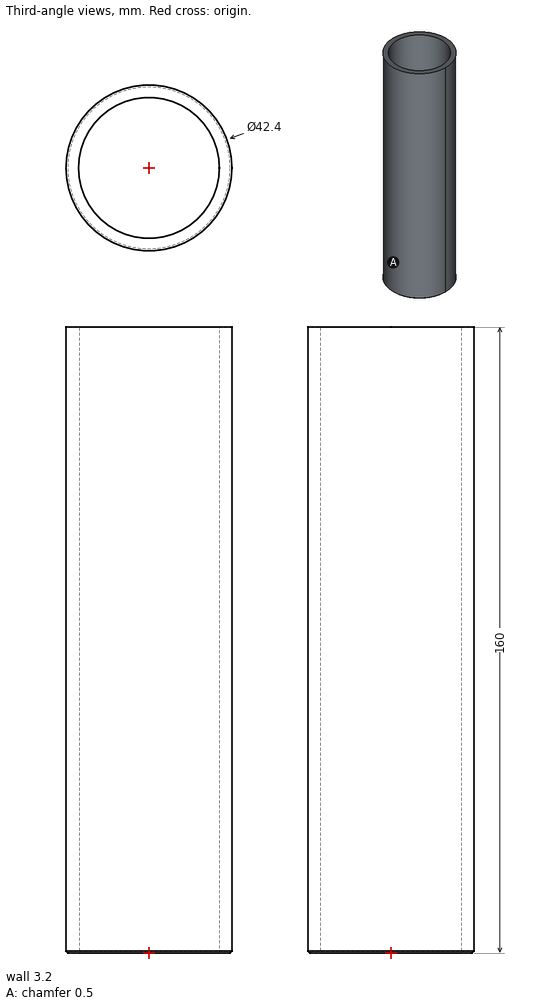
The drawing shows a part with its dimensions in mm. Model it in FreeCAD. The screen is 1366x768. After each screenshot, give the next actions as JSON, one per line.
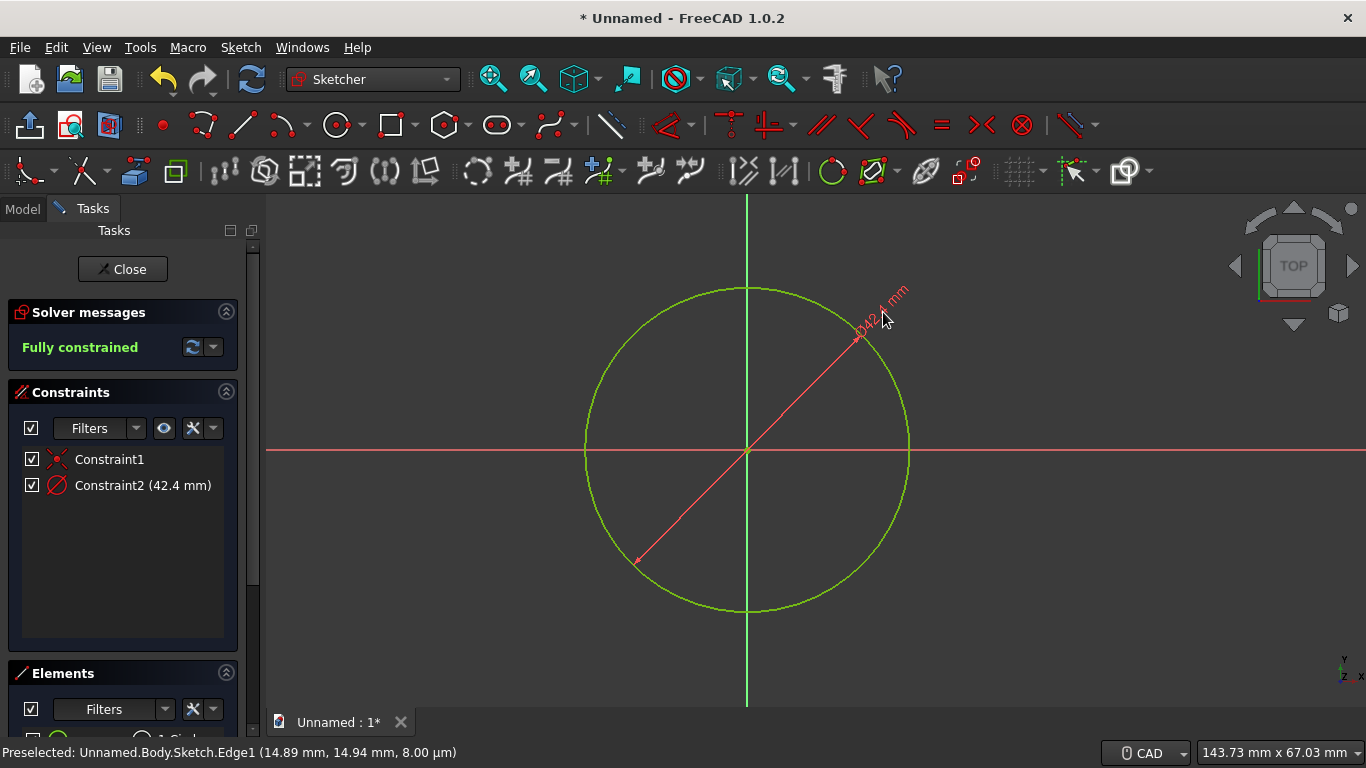
{"action": "left_click", "coordinate": [123, 269]}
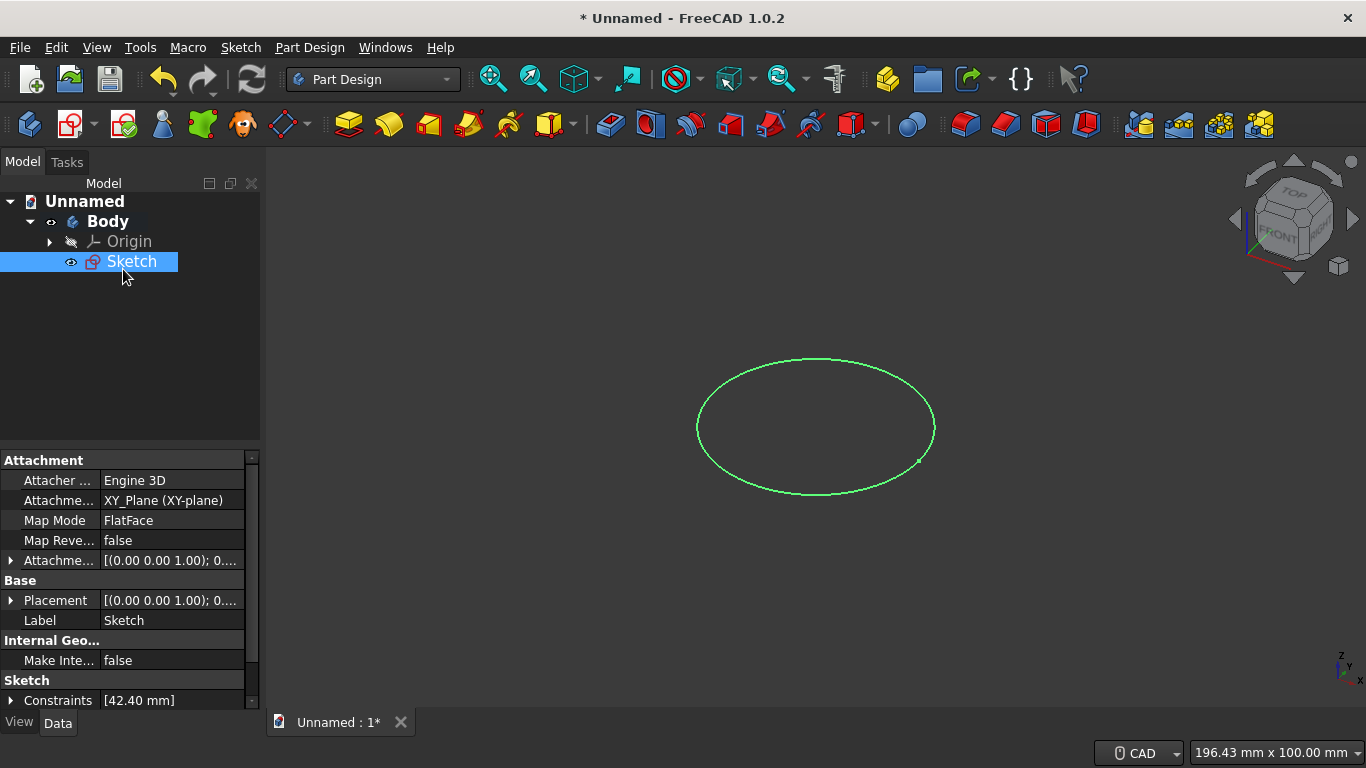
{"action": "left_click", "coordinate": [350, 124]}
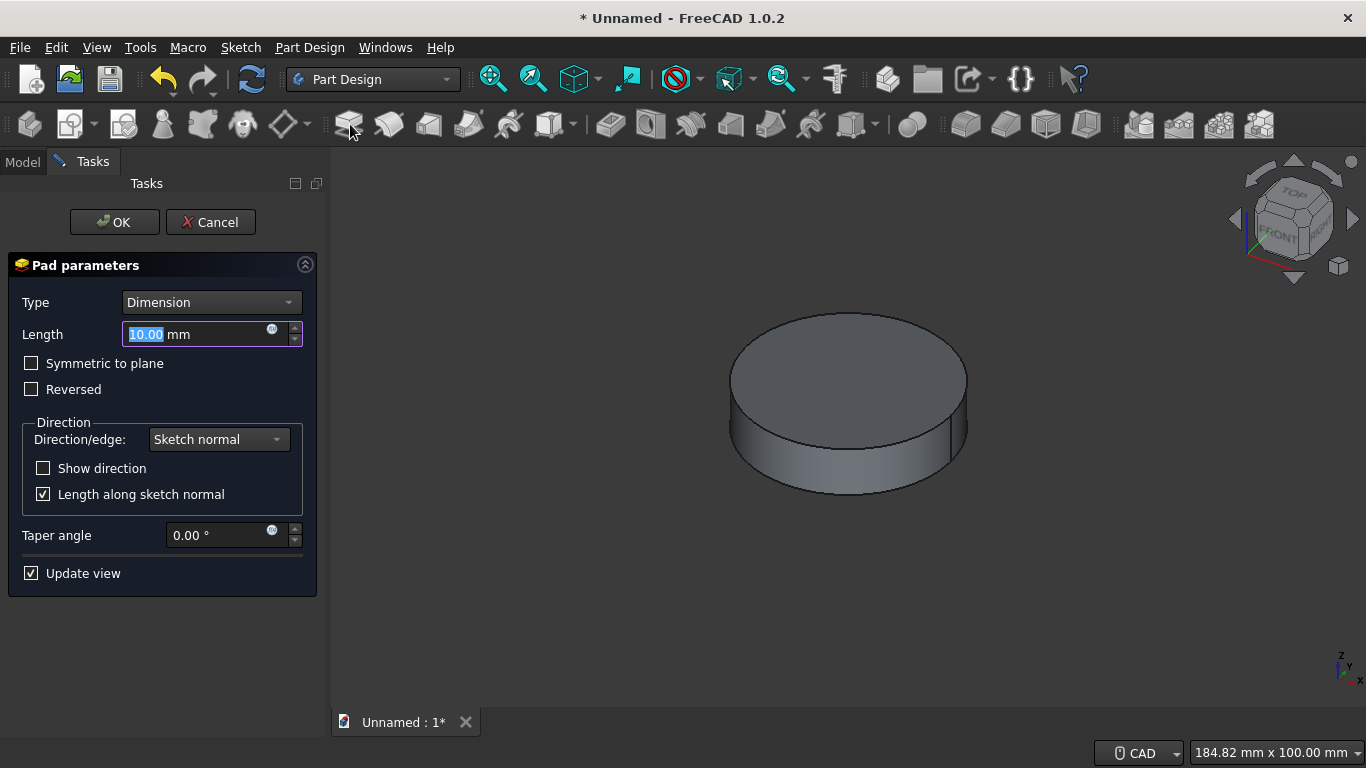
{"action": "type", "text": "160"}
{"action": "key", "text": "Tab"}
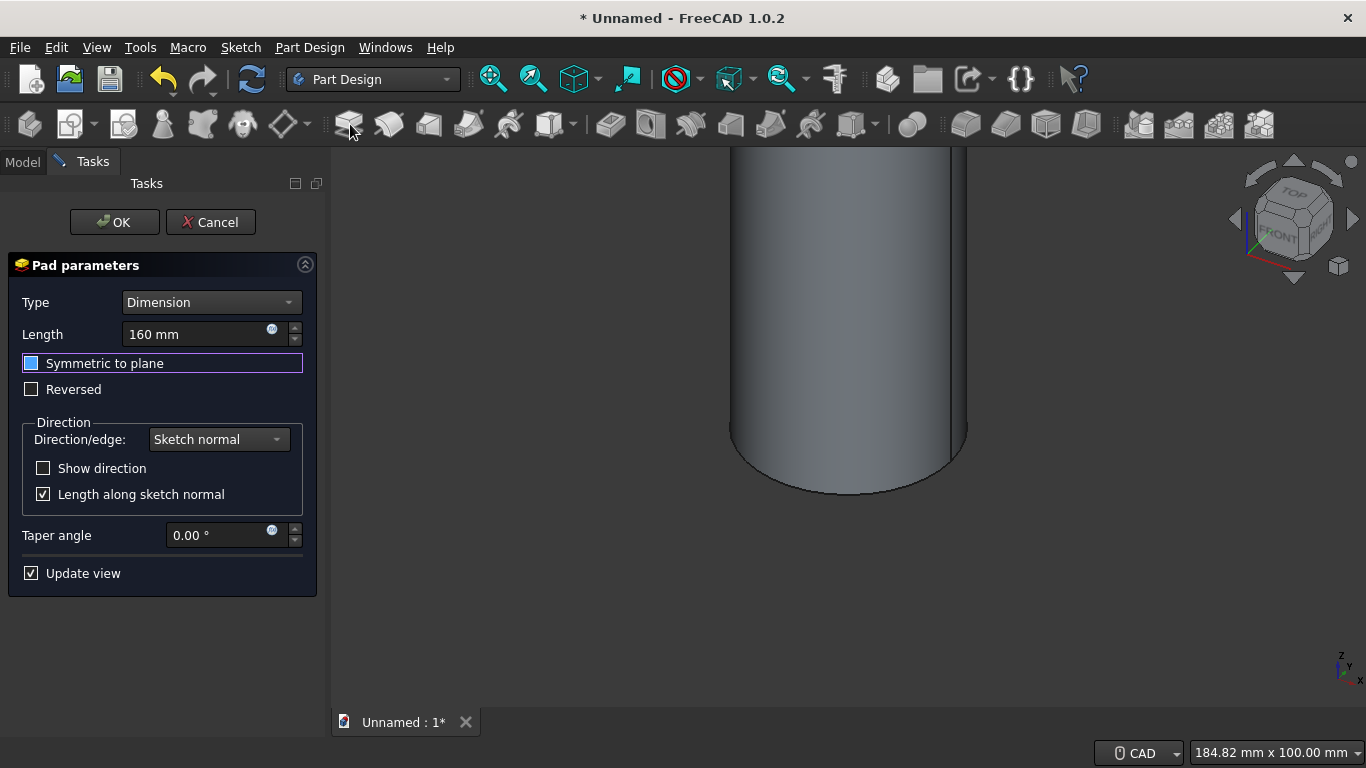
{"action": "left_click", "coordinate": [115, 222]}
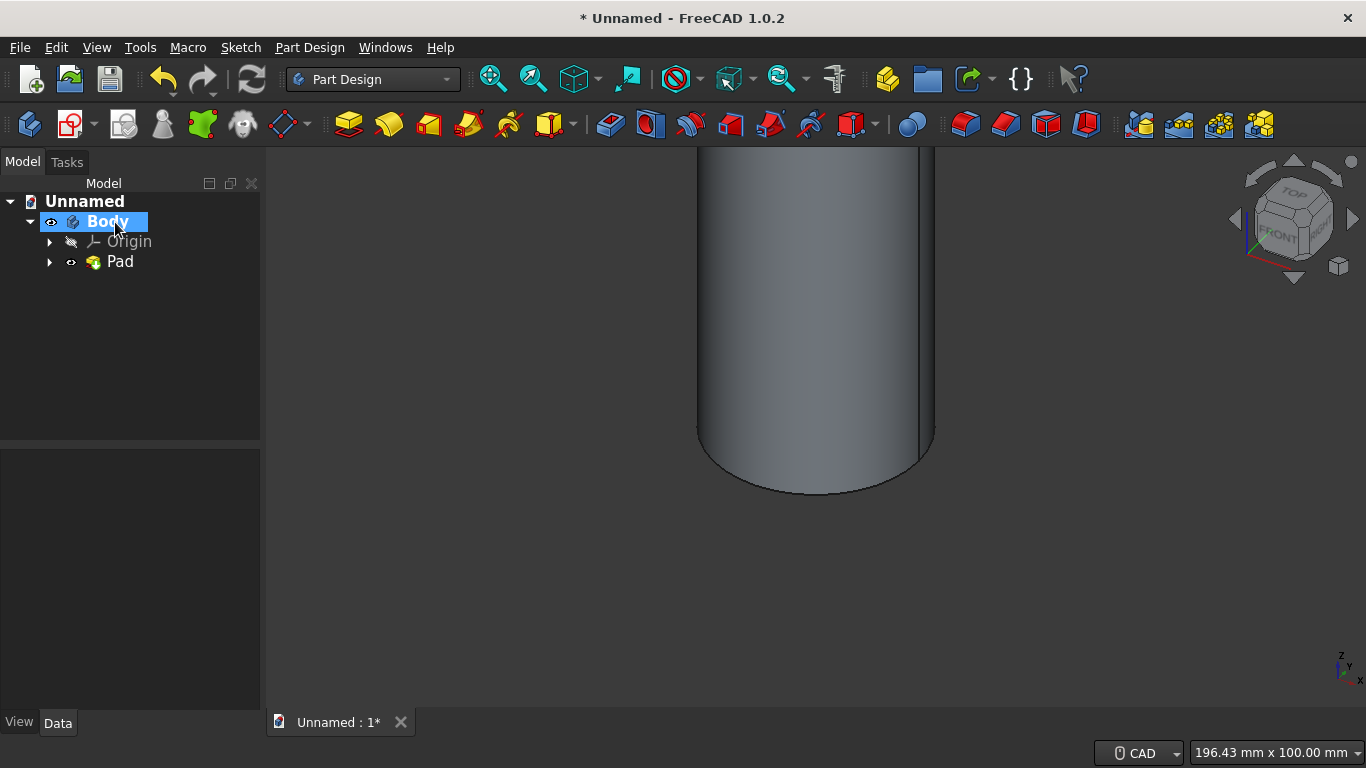
{"action": "left_click", "coordinate": [494, 80]}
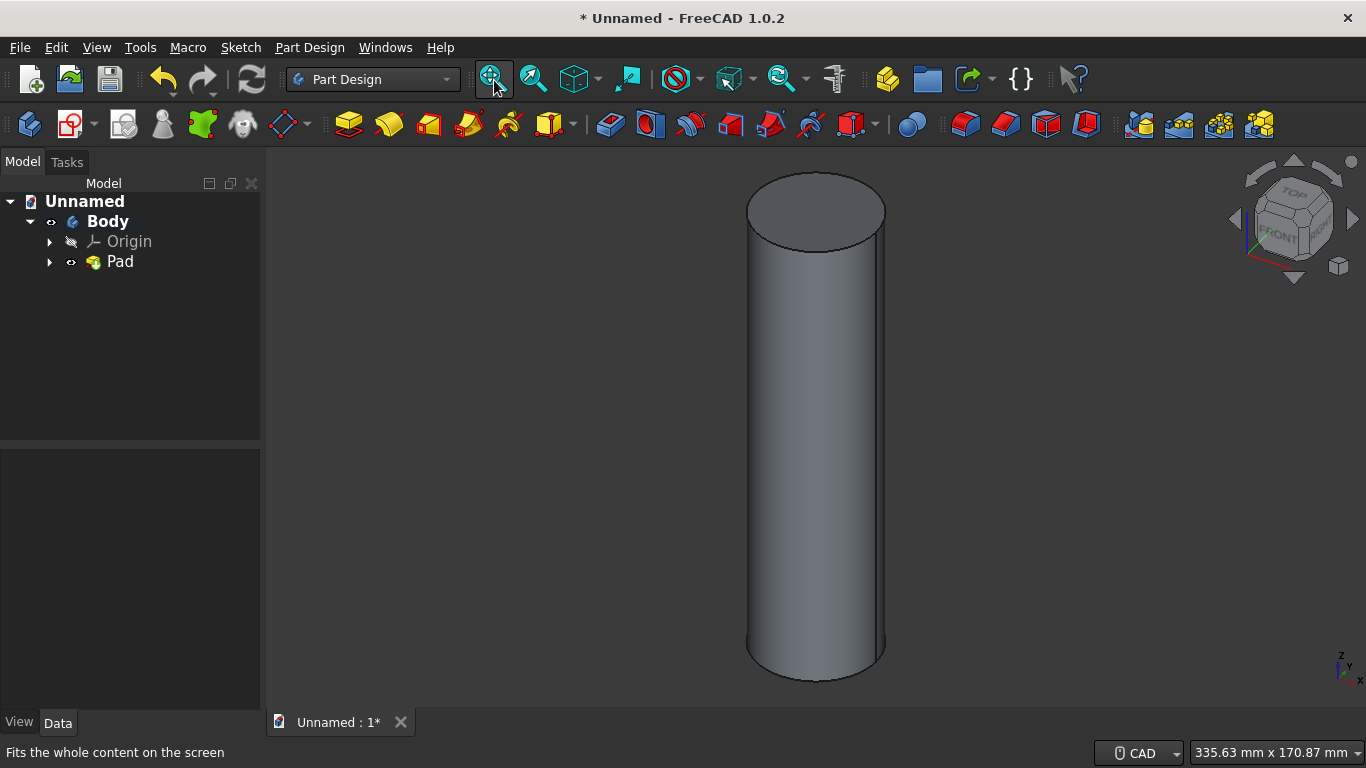
{"action": "left_click", "coordinate": [816, 211]}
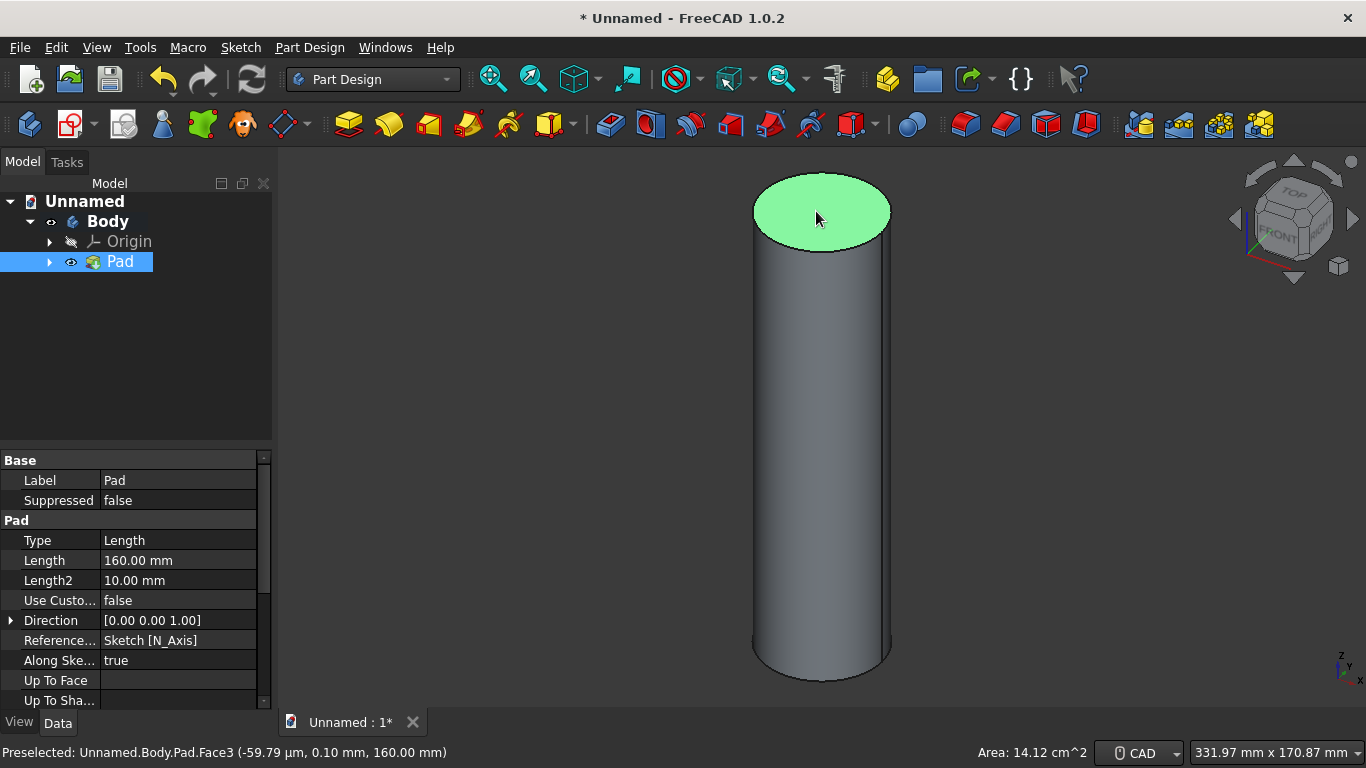
{"action": "key", "text": "0"}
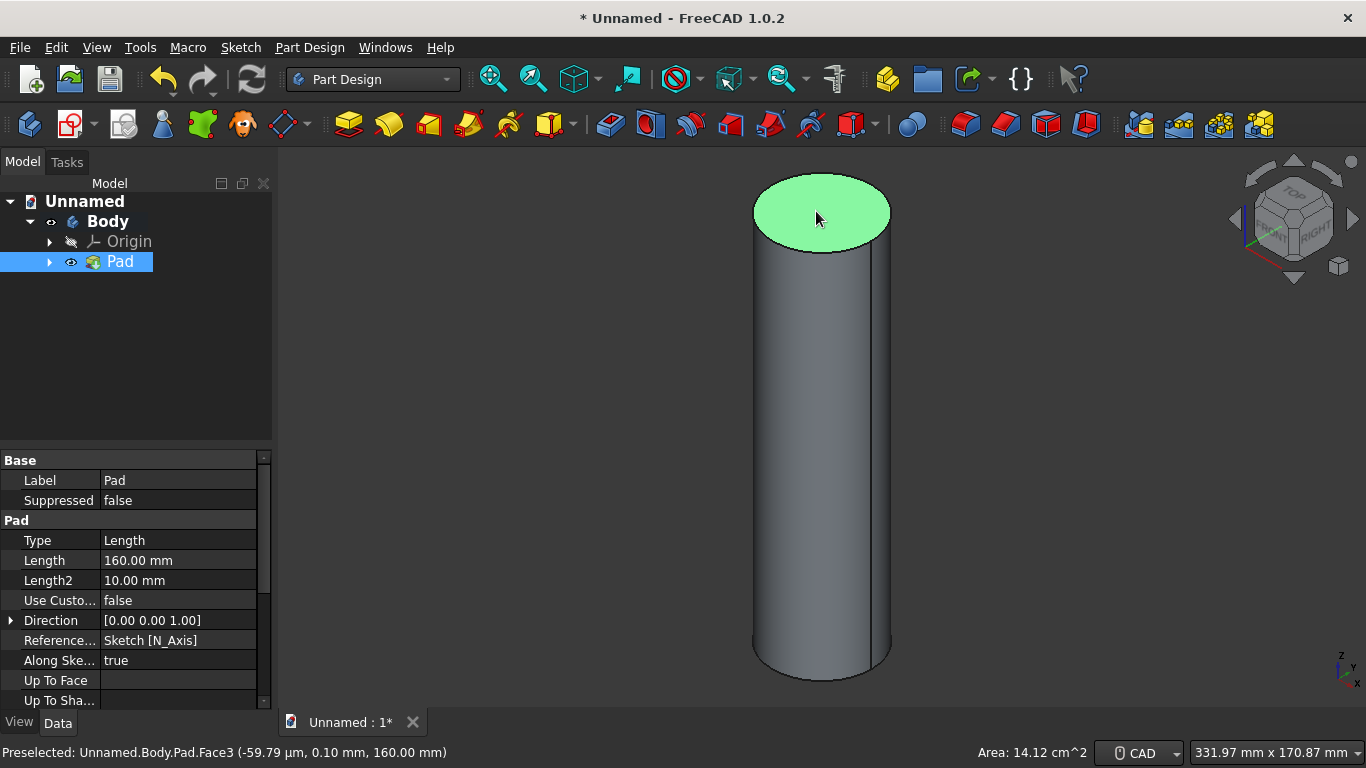
{"action": "key", "text": "2"}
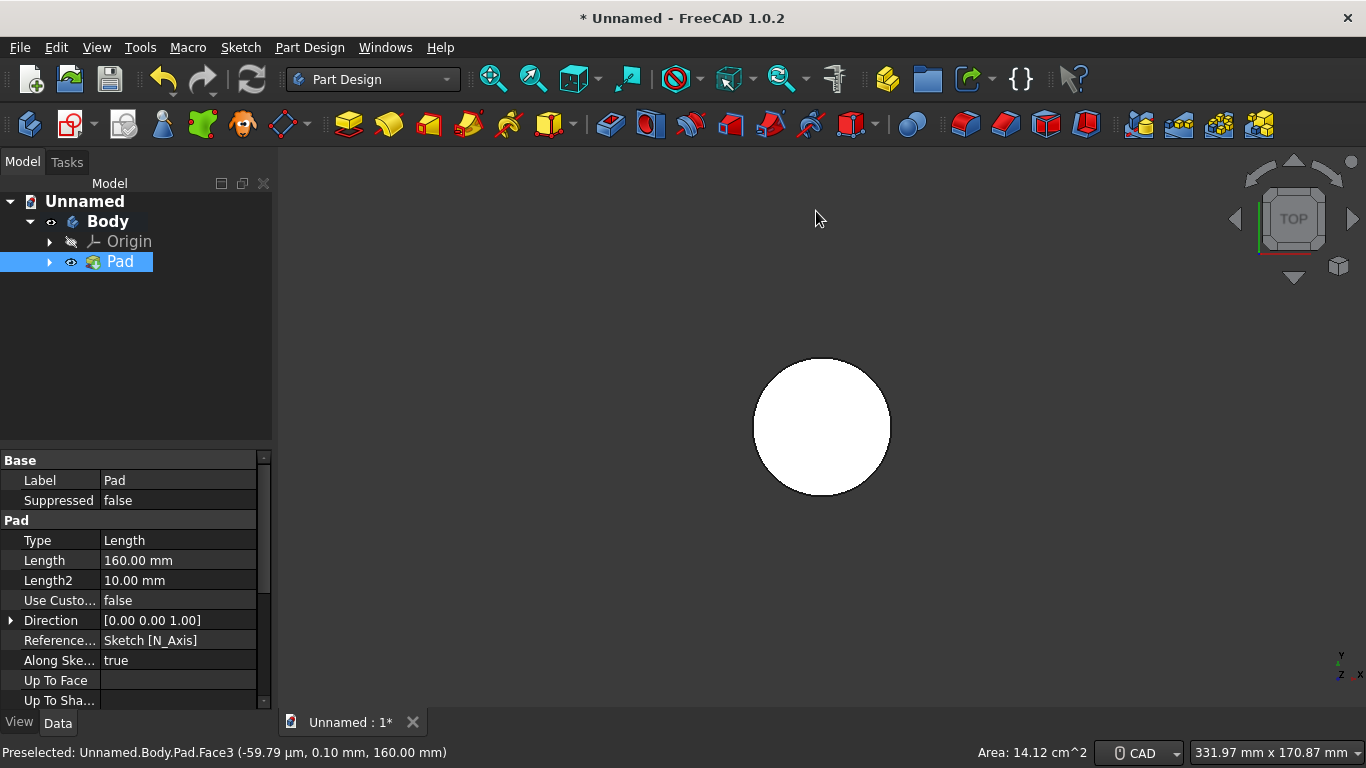
{"action": "left_click", "coordinate": [494, 80]}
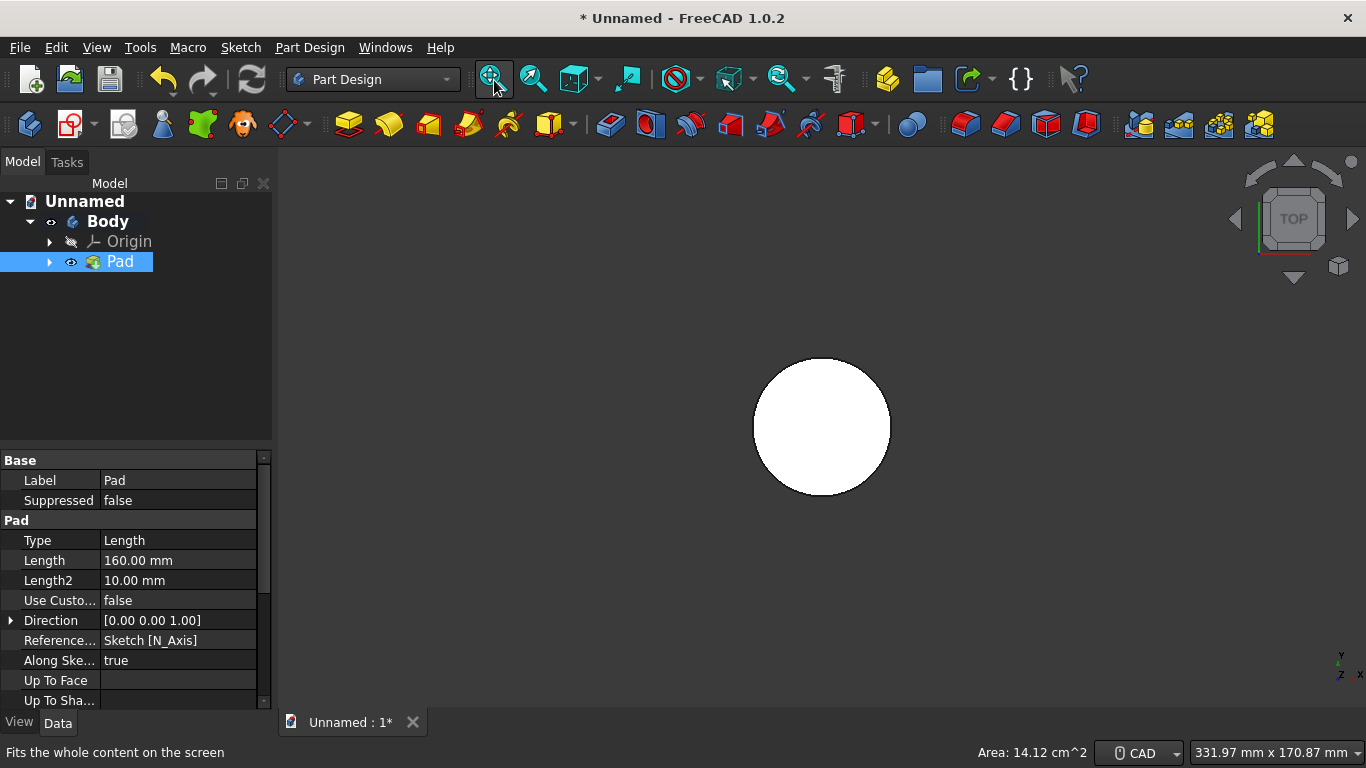
{"action": "key", "text": "1"}